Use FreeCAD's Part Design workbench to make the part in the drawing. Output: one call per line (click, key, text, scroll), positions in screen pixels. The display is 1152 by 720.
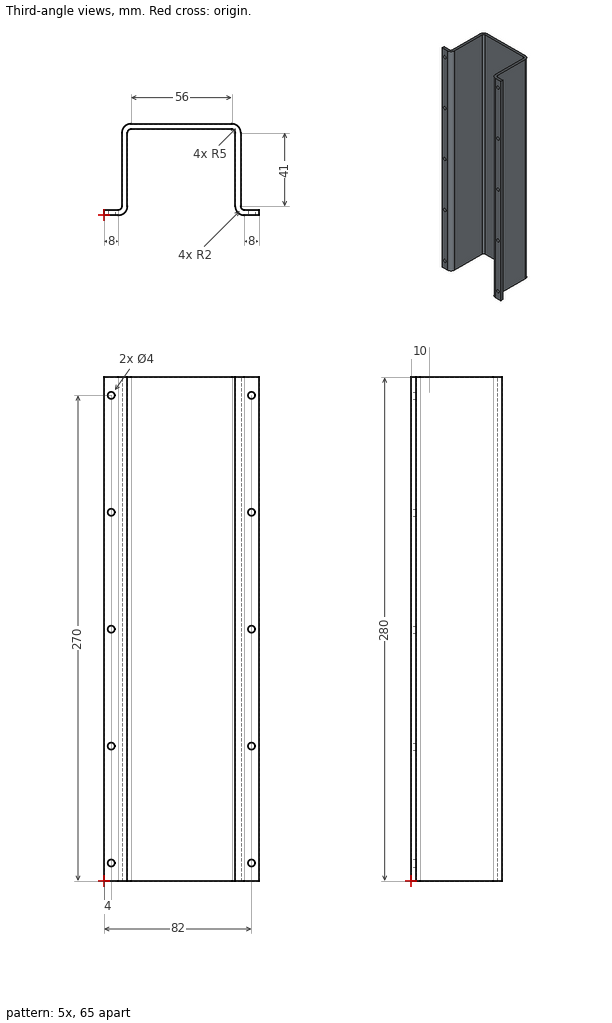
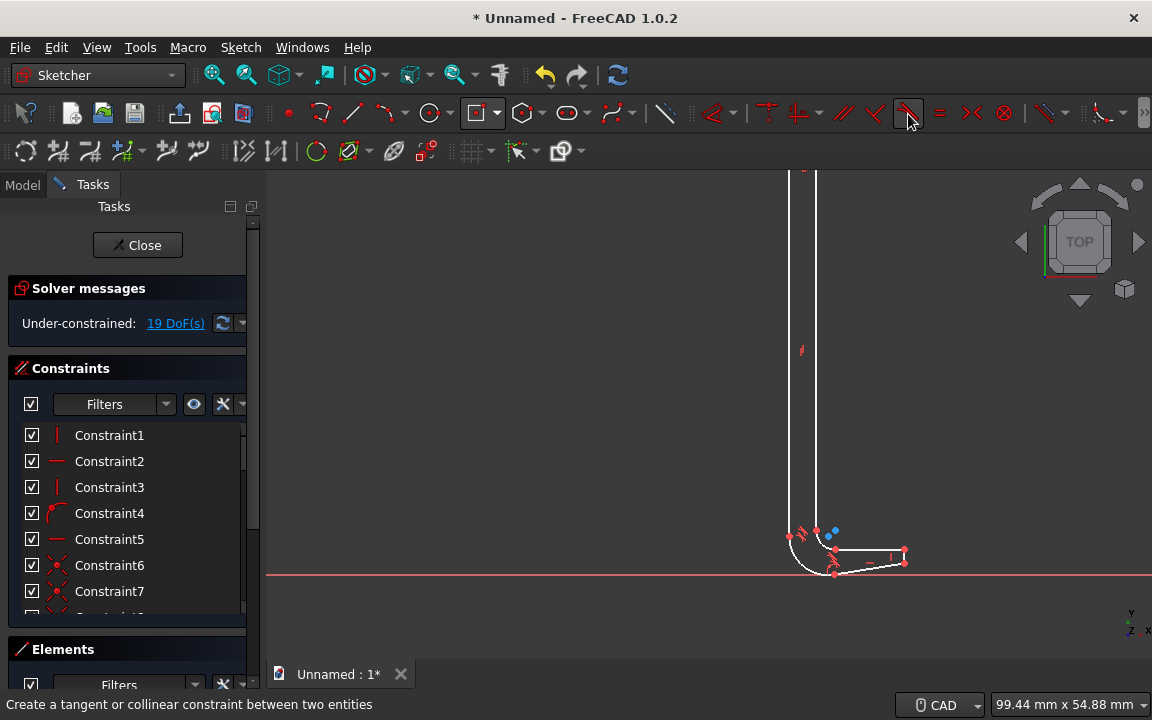
scroll(882, 551, down, 2)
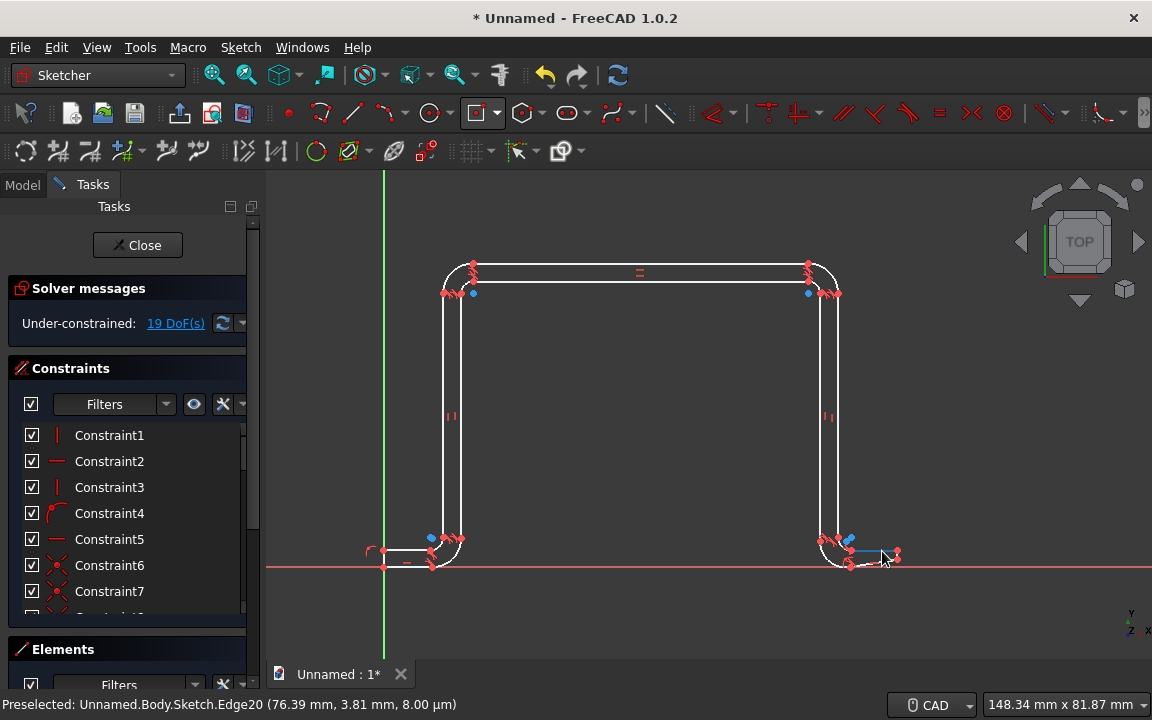
click(398, 567)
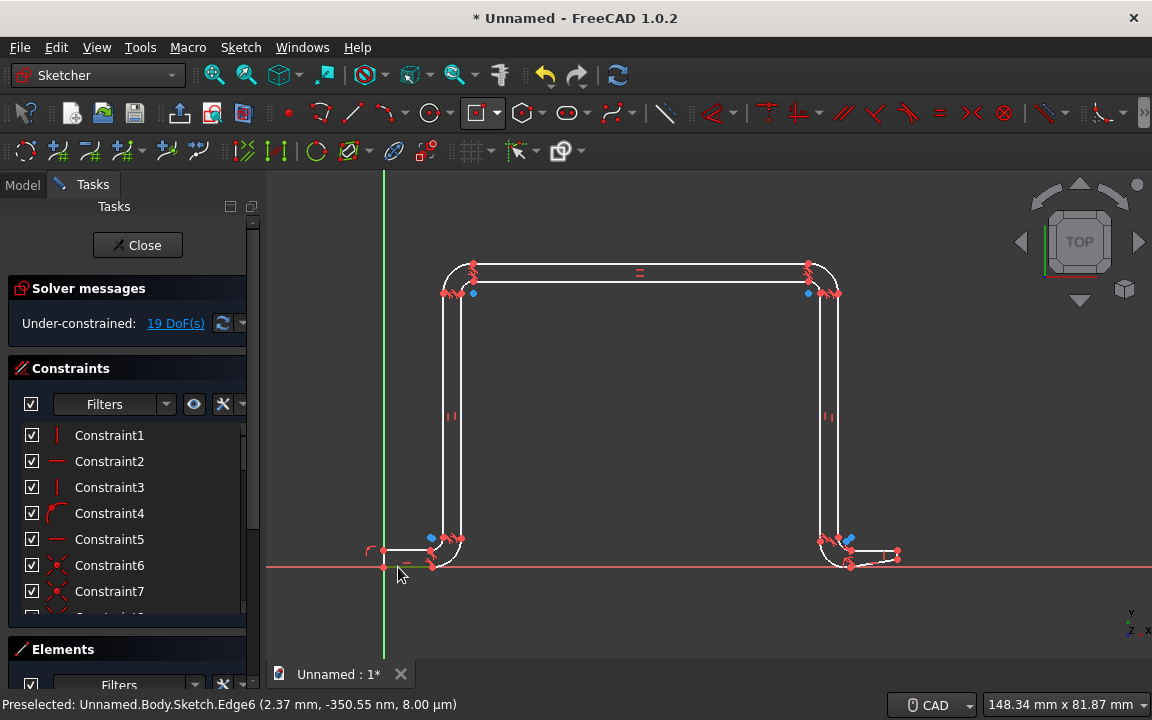
key(h)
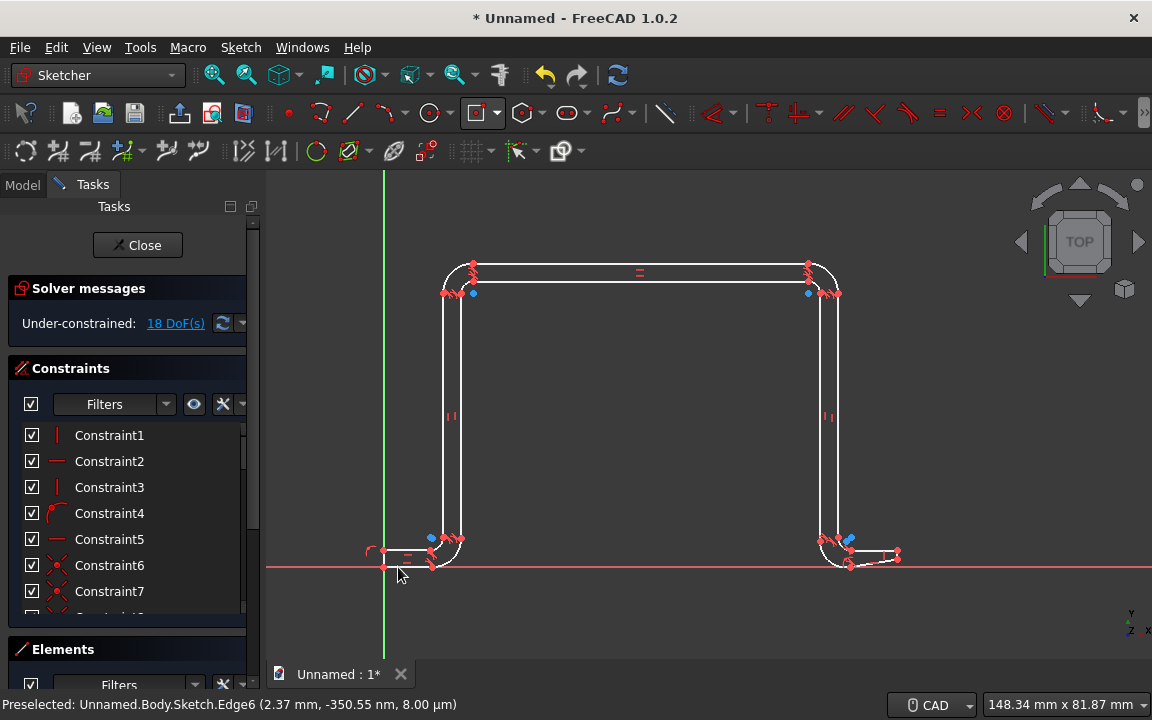
click(864, 565)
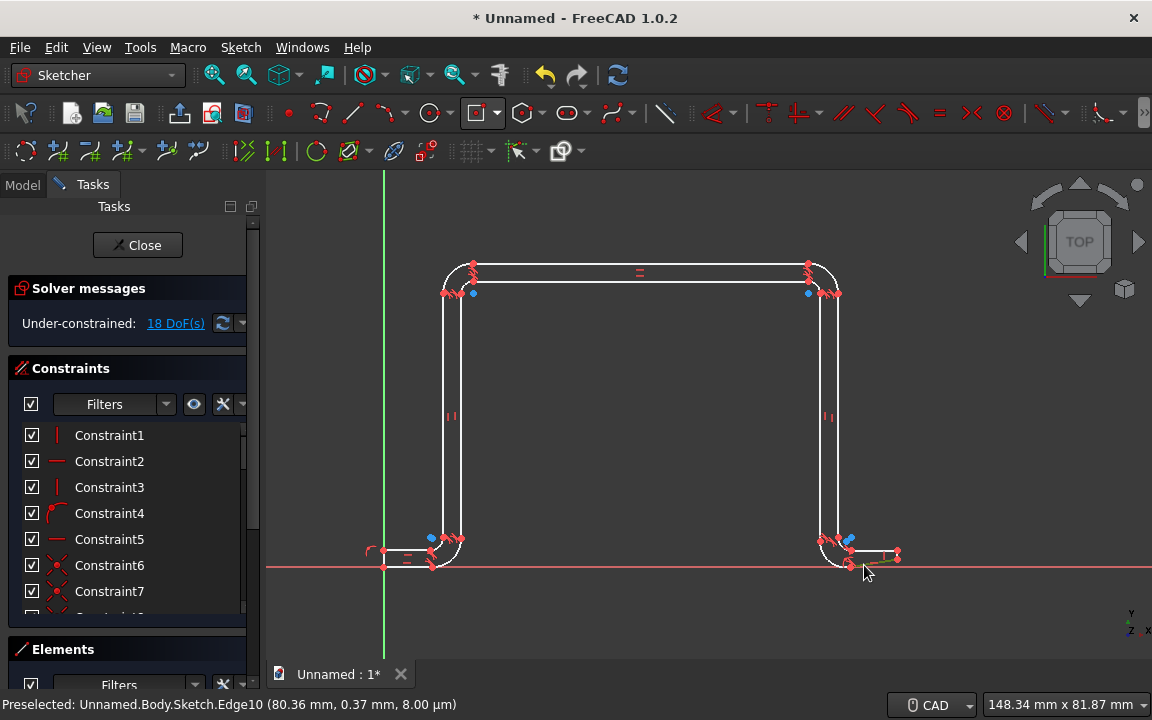
key(h)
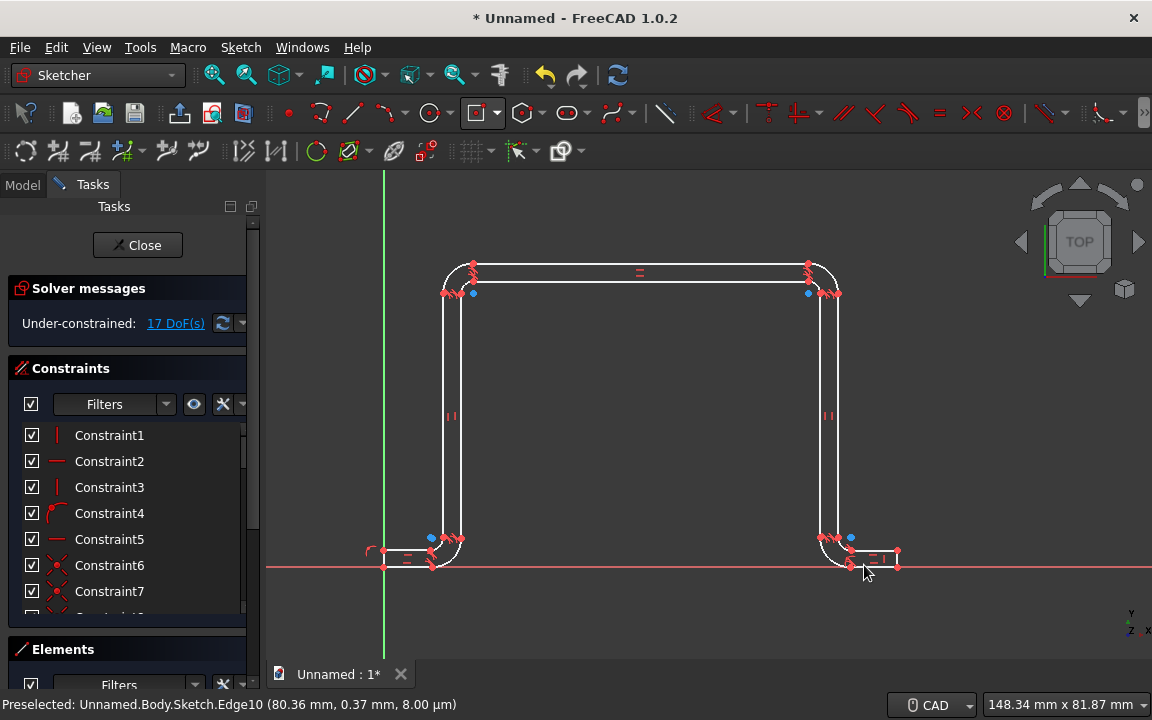
scroll(439, 547, up, 2)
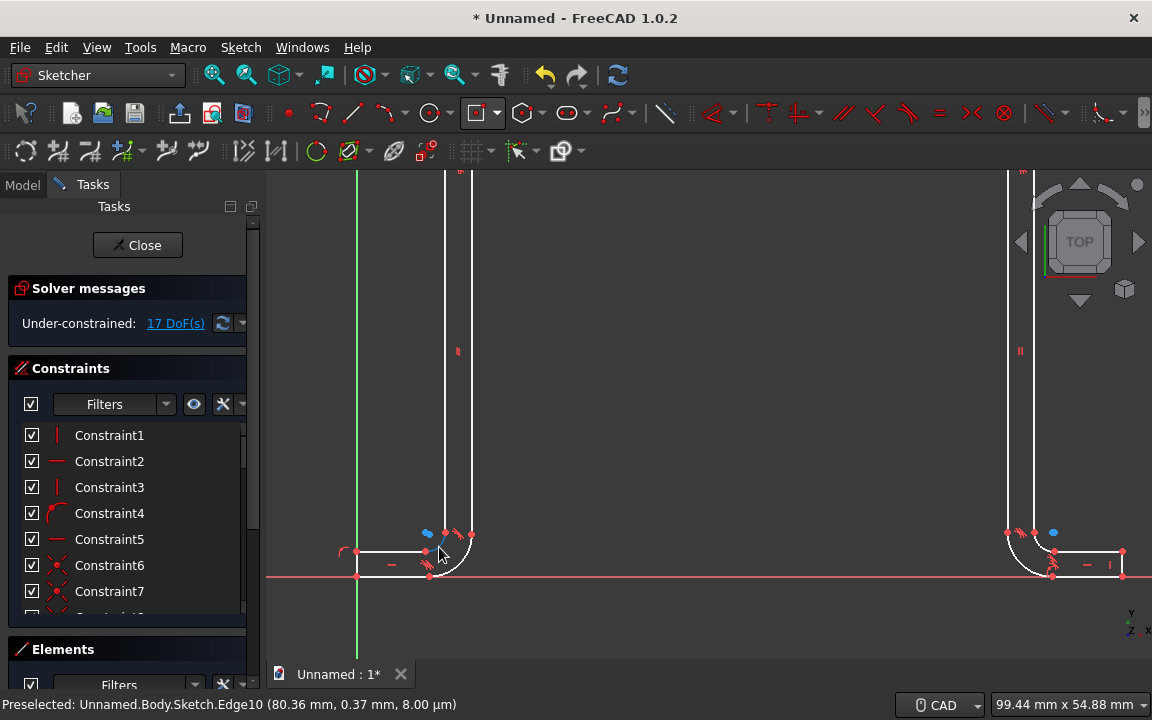
click(439, 546)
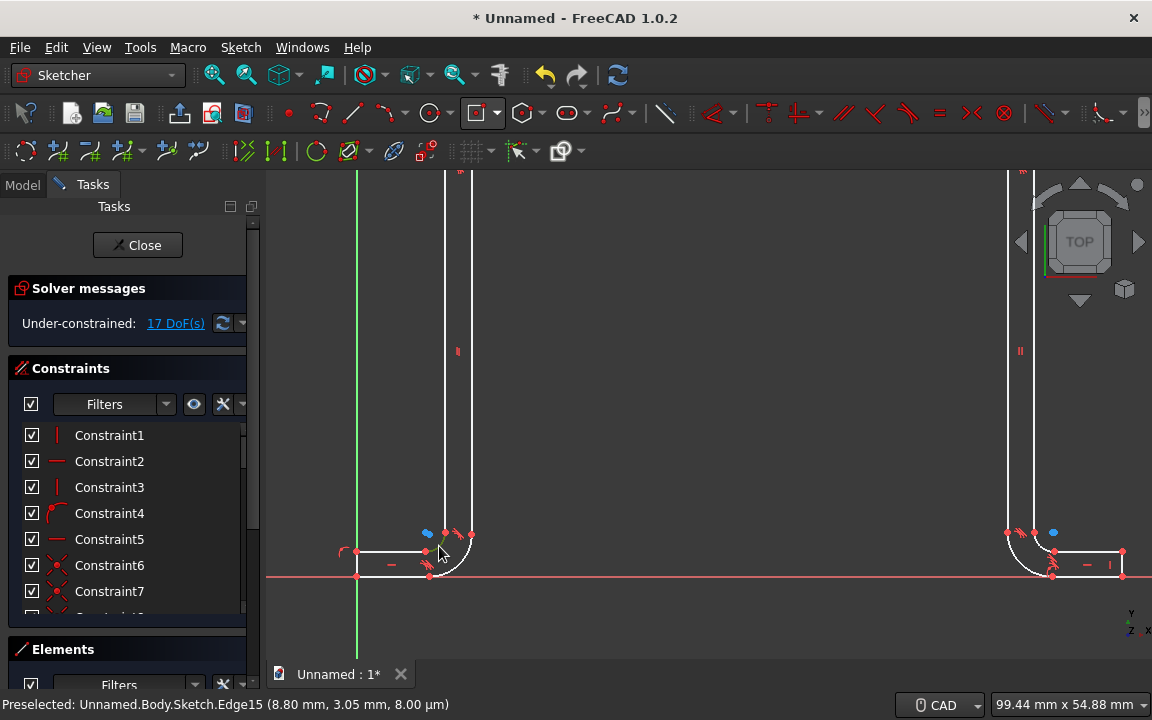
click(467, 553)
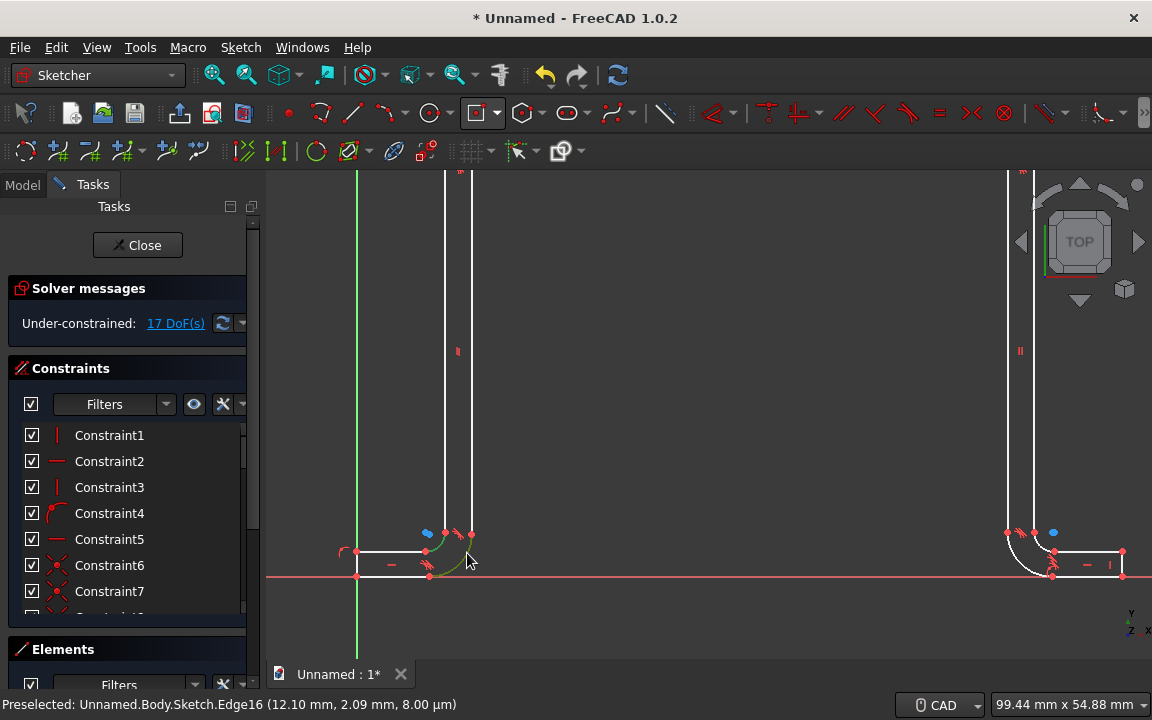
key(c)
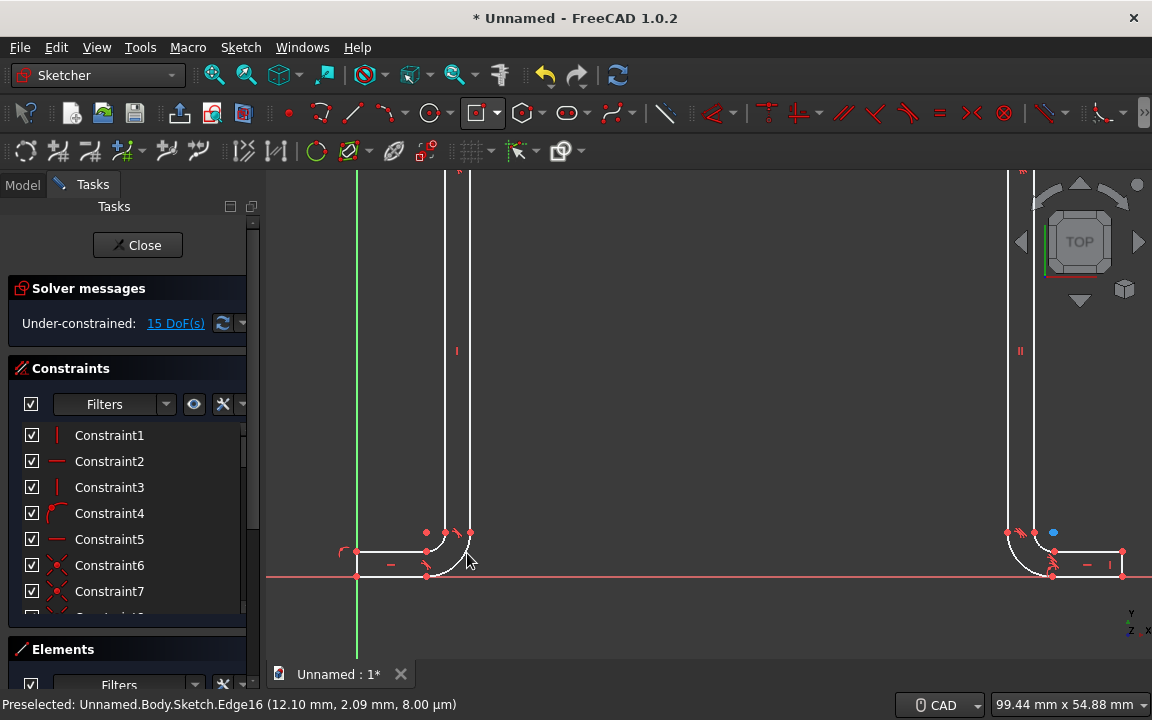
scroll(439, 547, down, 2)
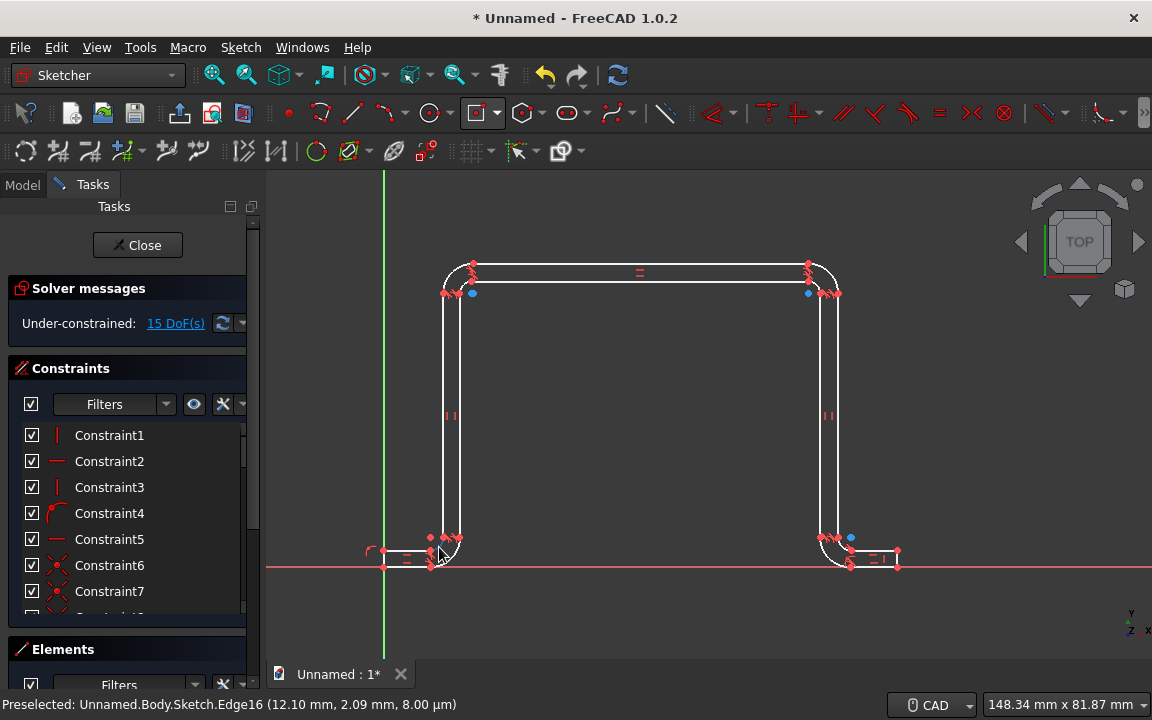
click(460, 267)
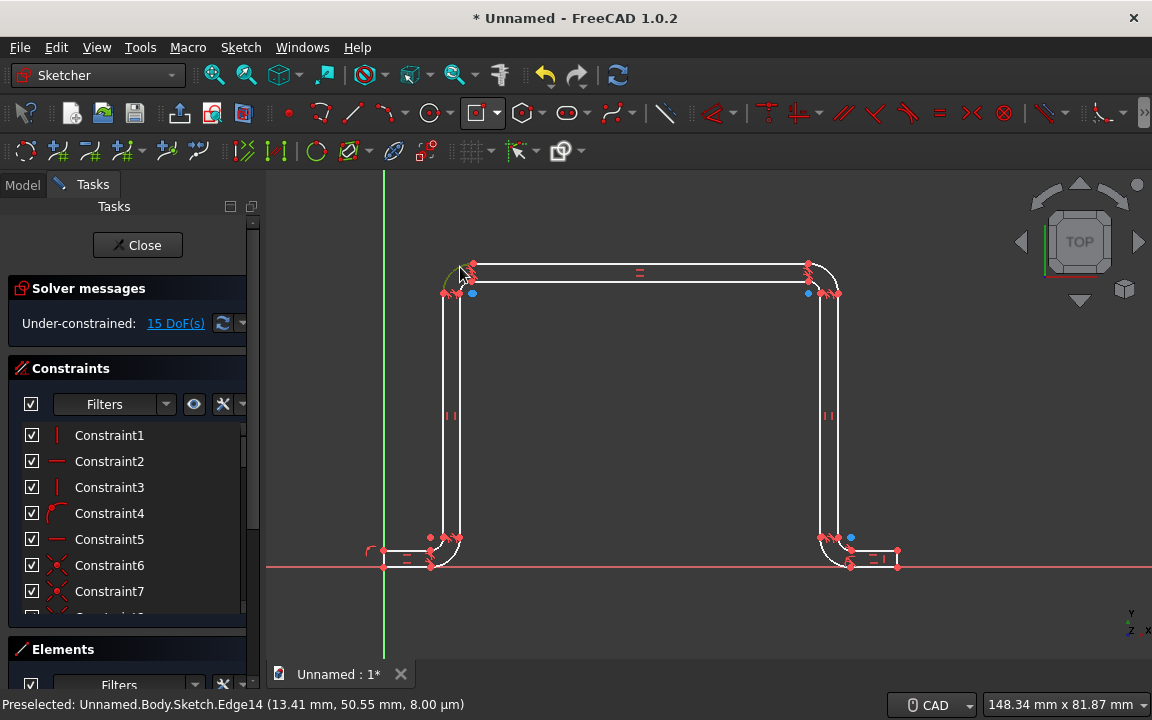
scroll(463, 285, up, 3)